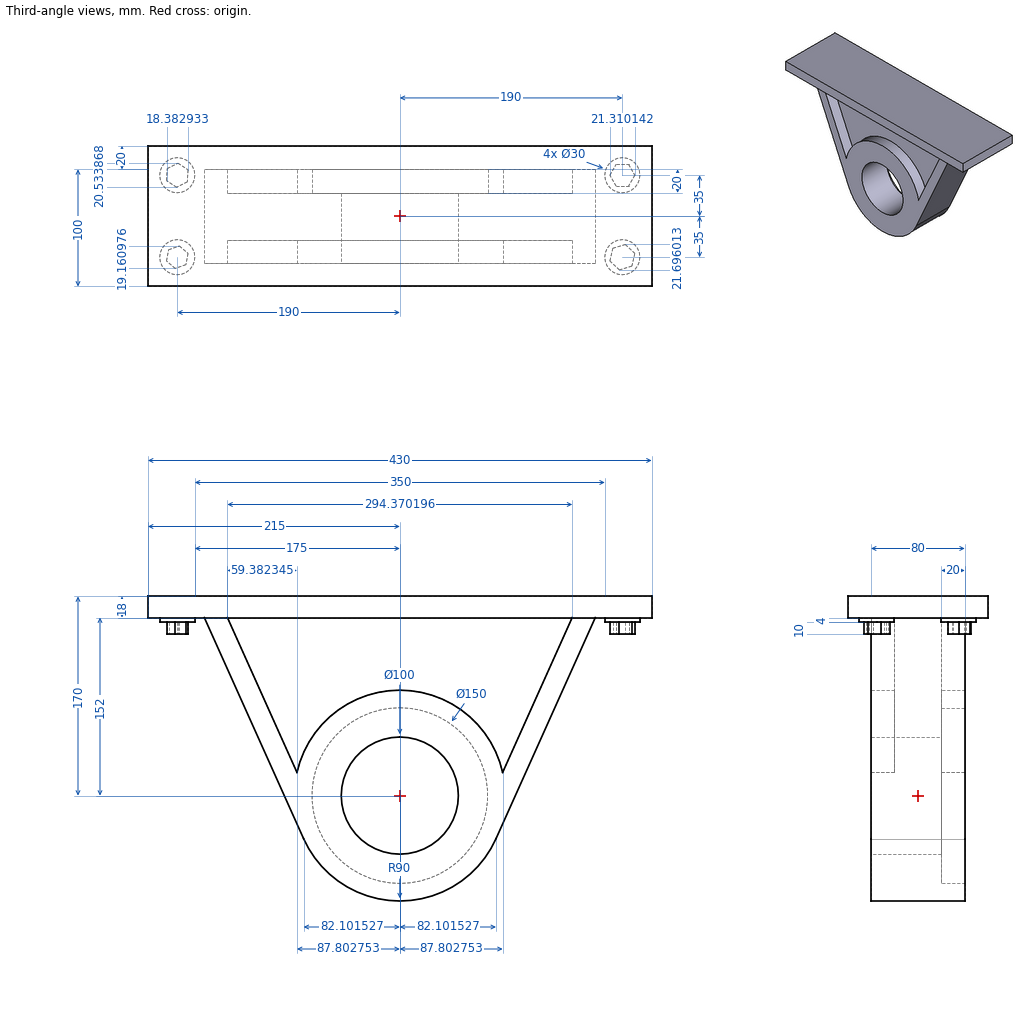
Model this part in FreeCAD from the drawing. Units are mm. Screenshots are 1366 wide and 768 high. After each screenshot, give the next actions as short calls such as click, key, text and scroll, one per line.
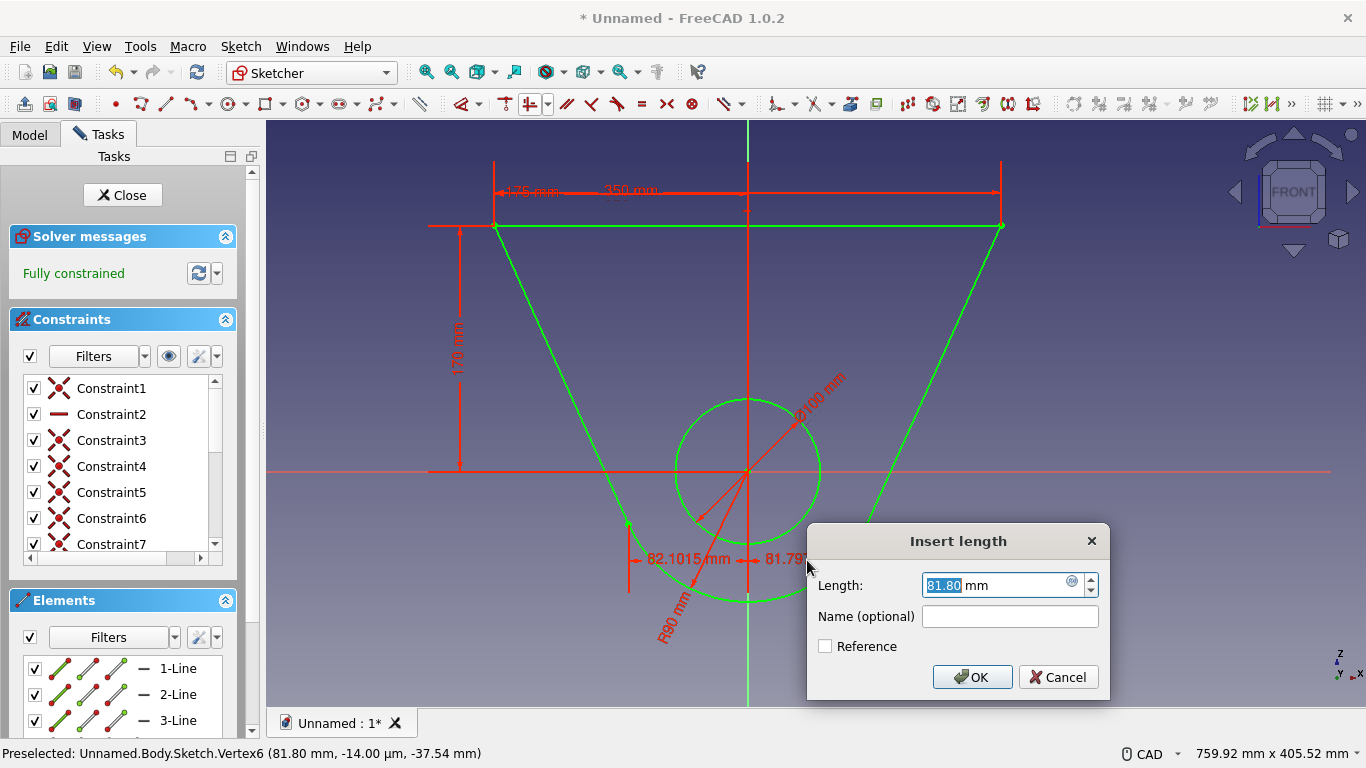
text(82.101527)
key(Return)
key(Escape)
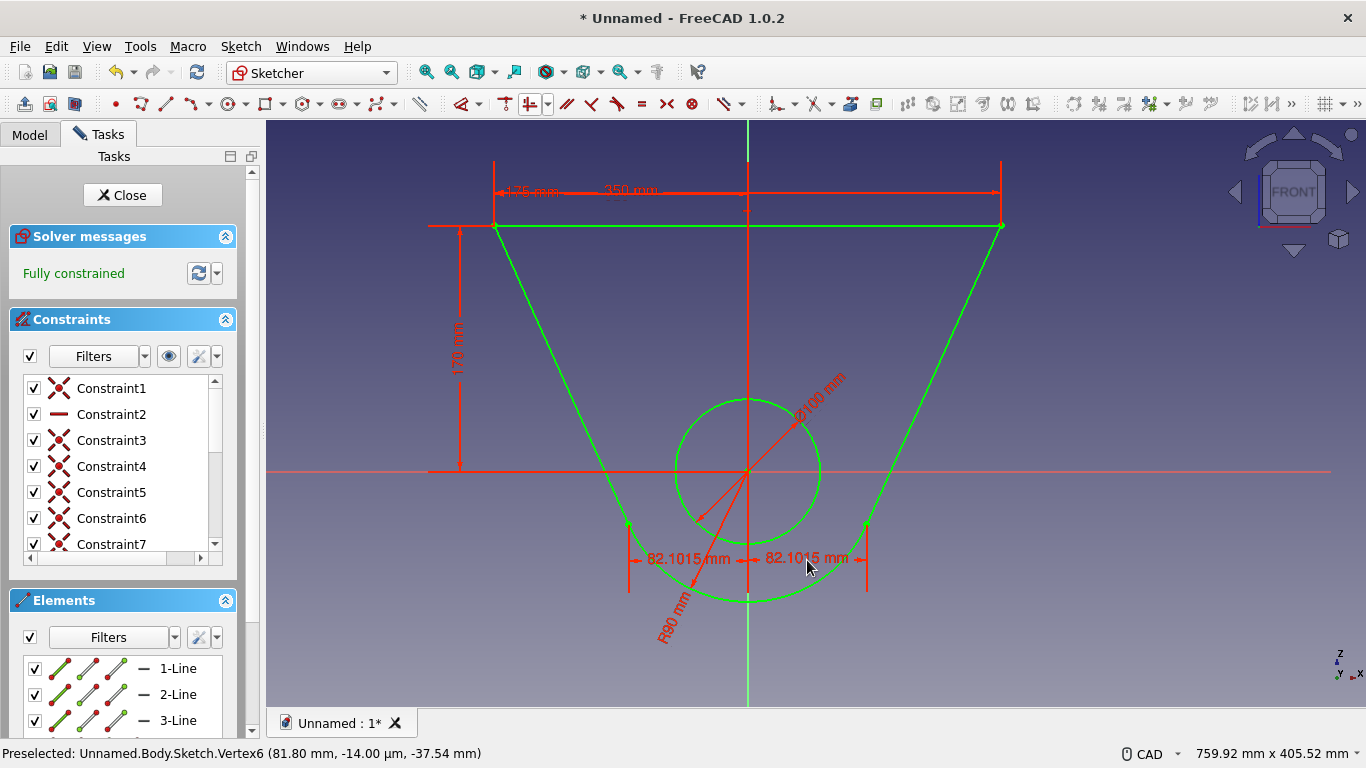
click(123, 195)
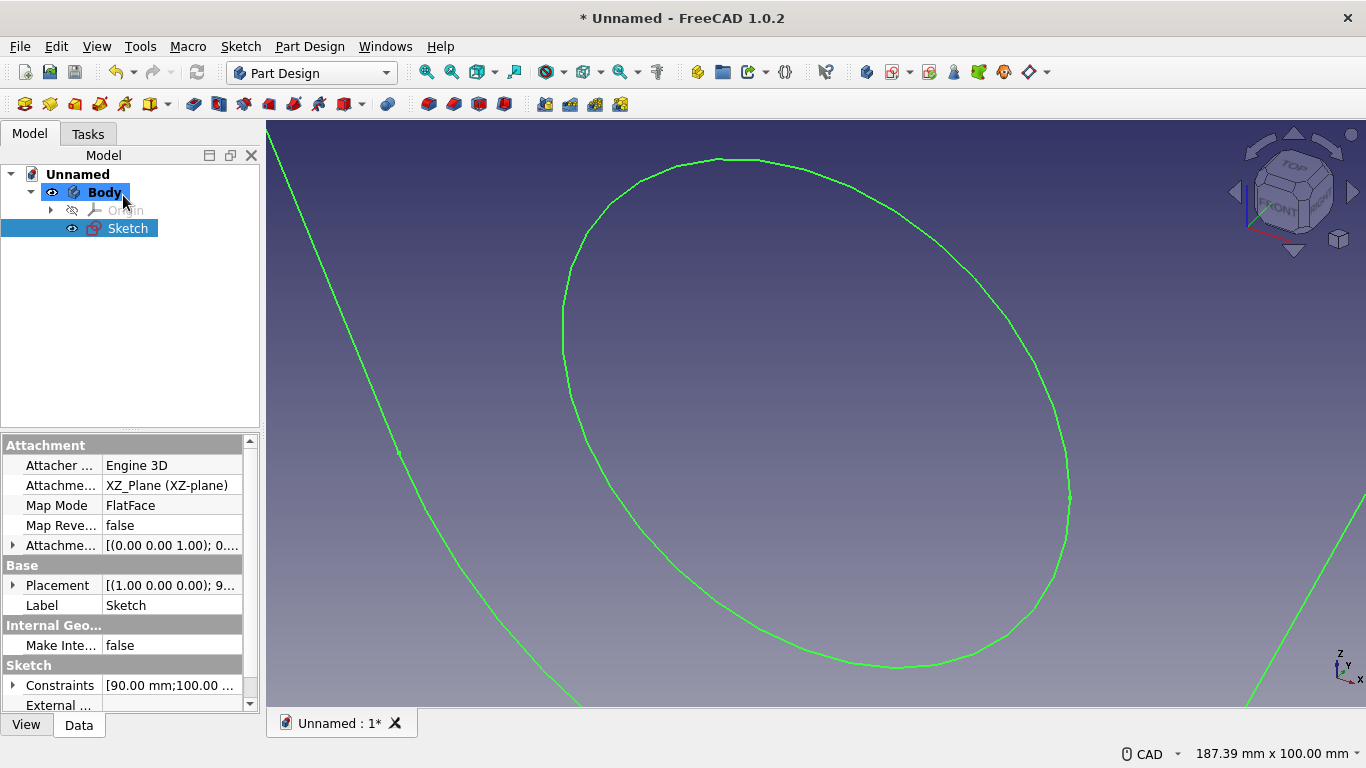
click(25, 104)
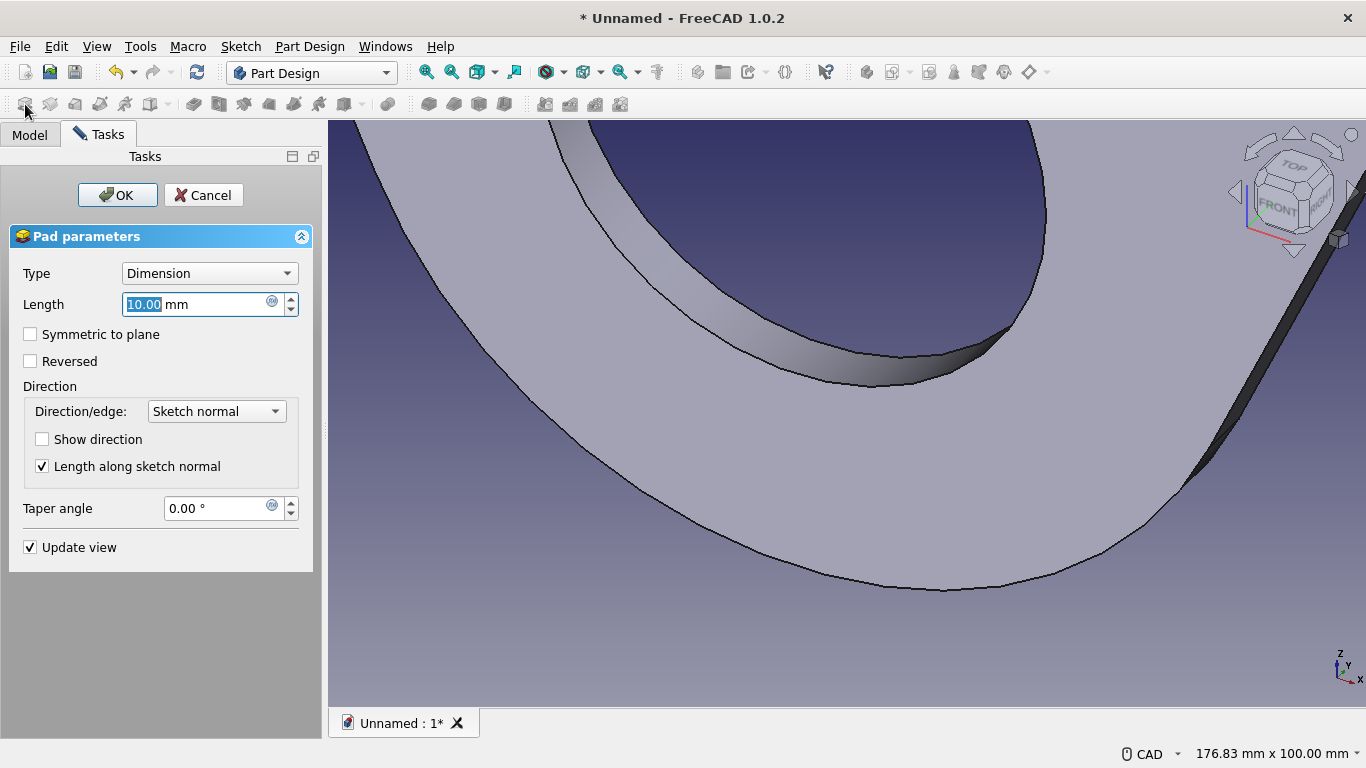
text(80)
key(Tab)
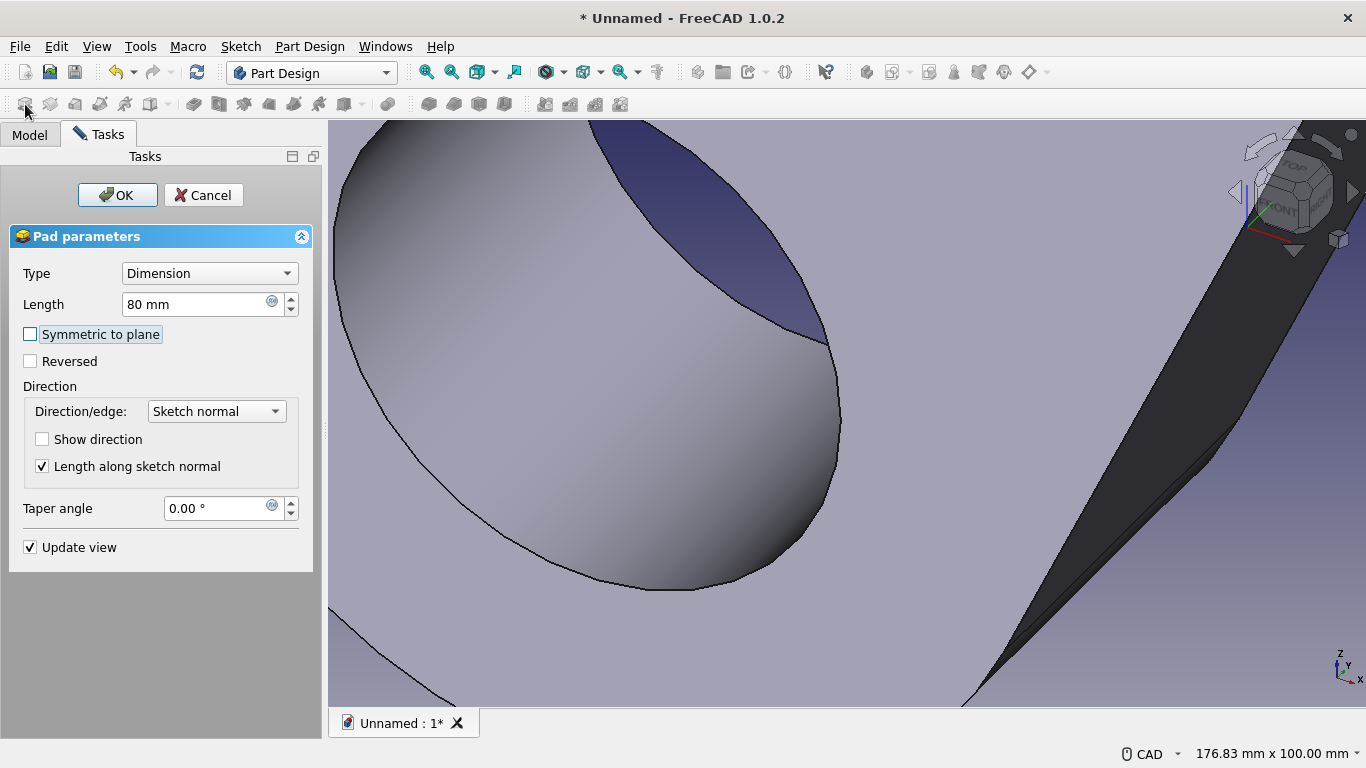
click(31, 334)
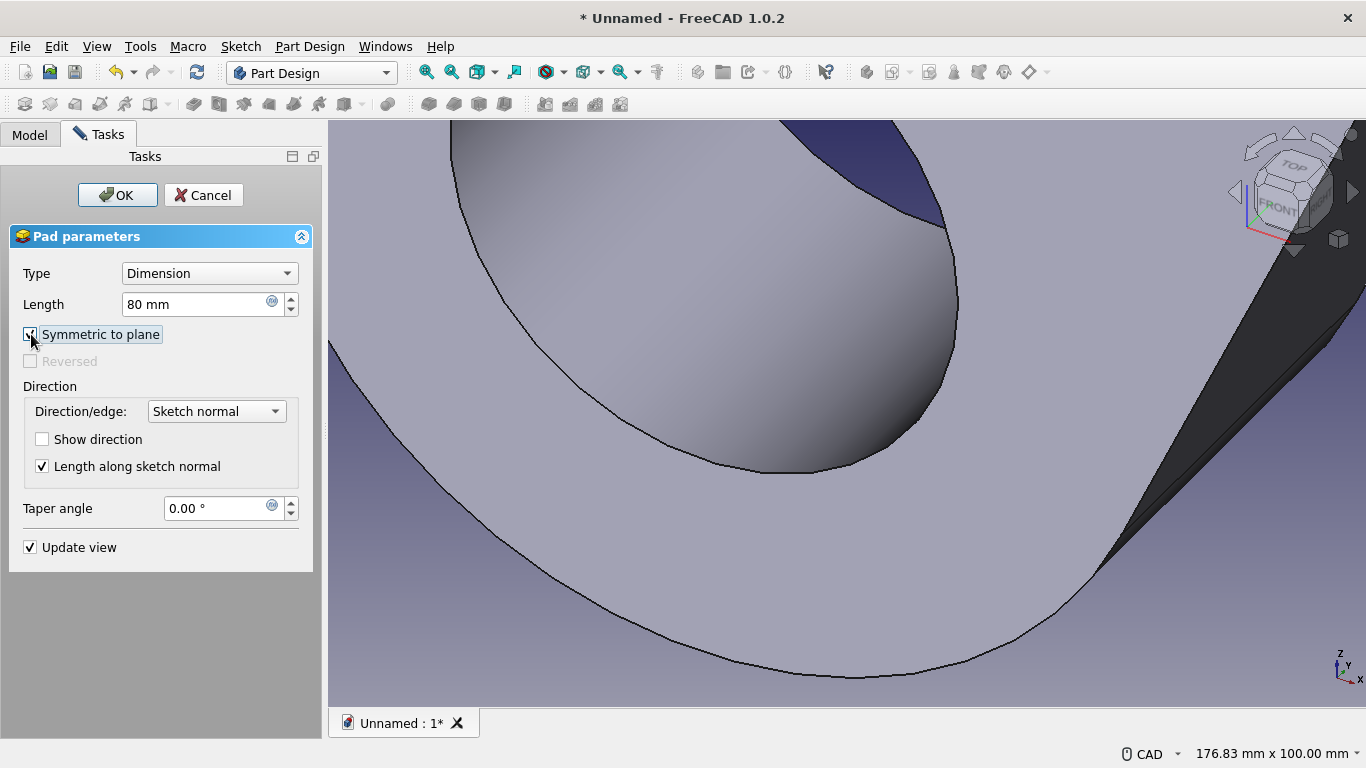
click(118, 195)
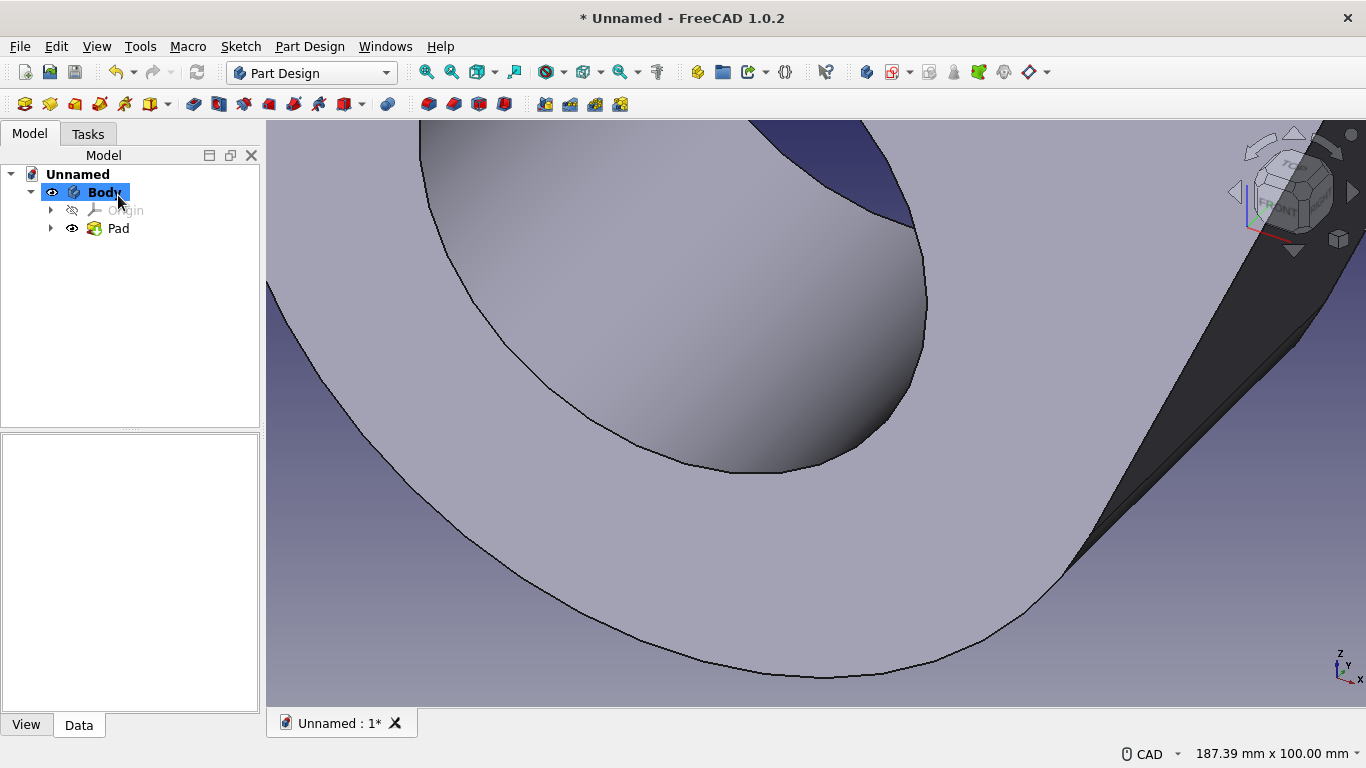
click(427, 72)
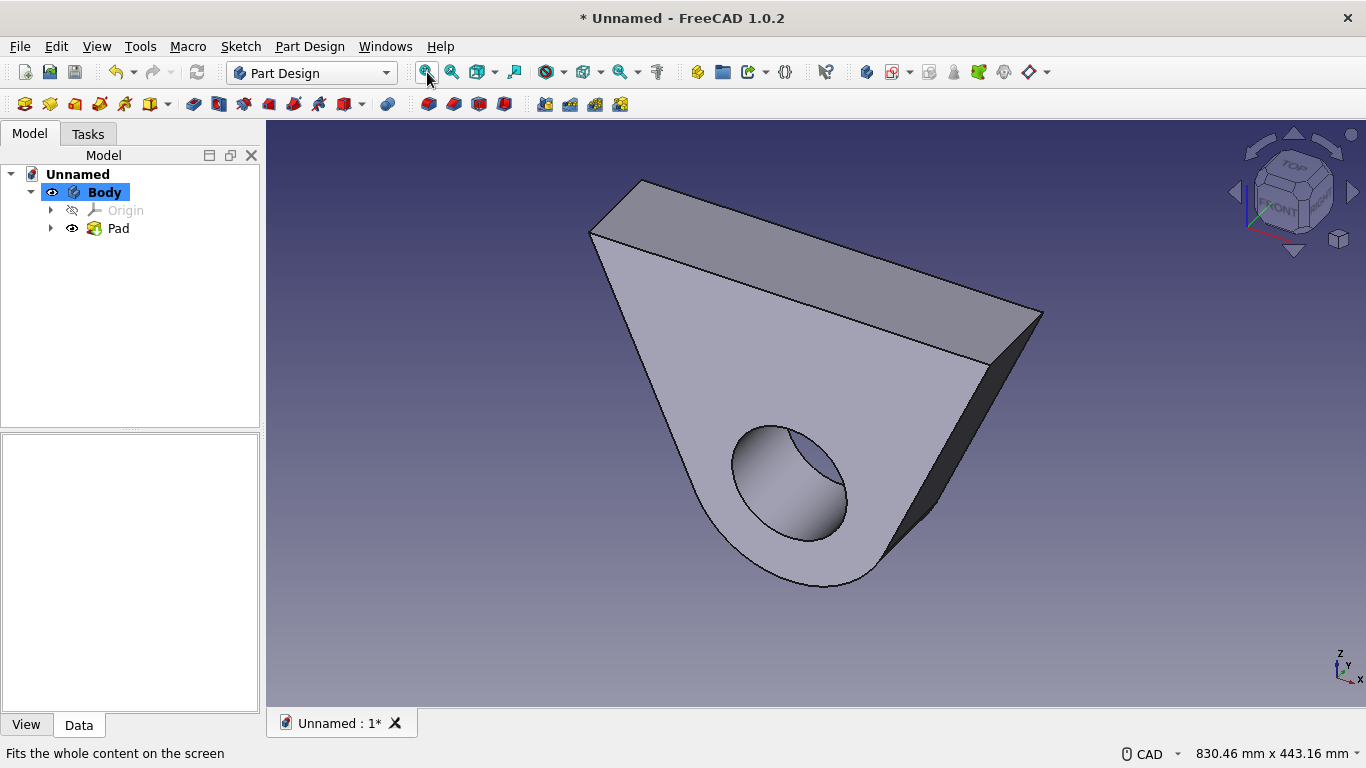
click(51, 210)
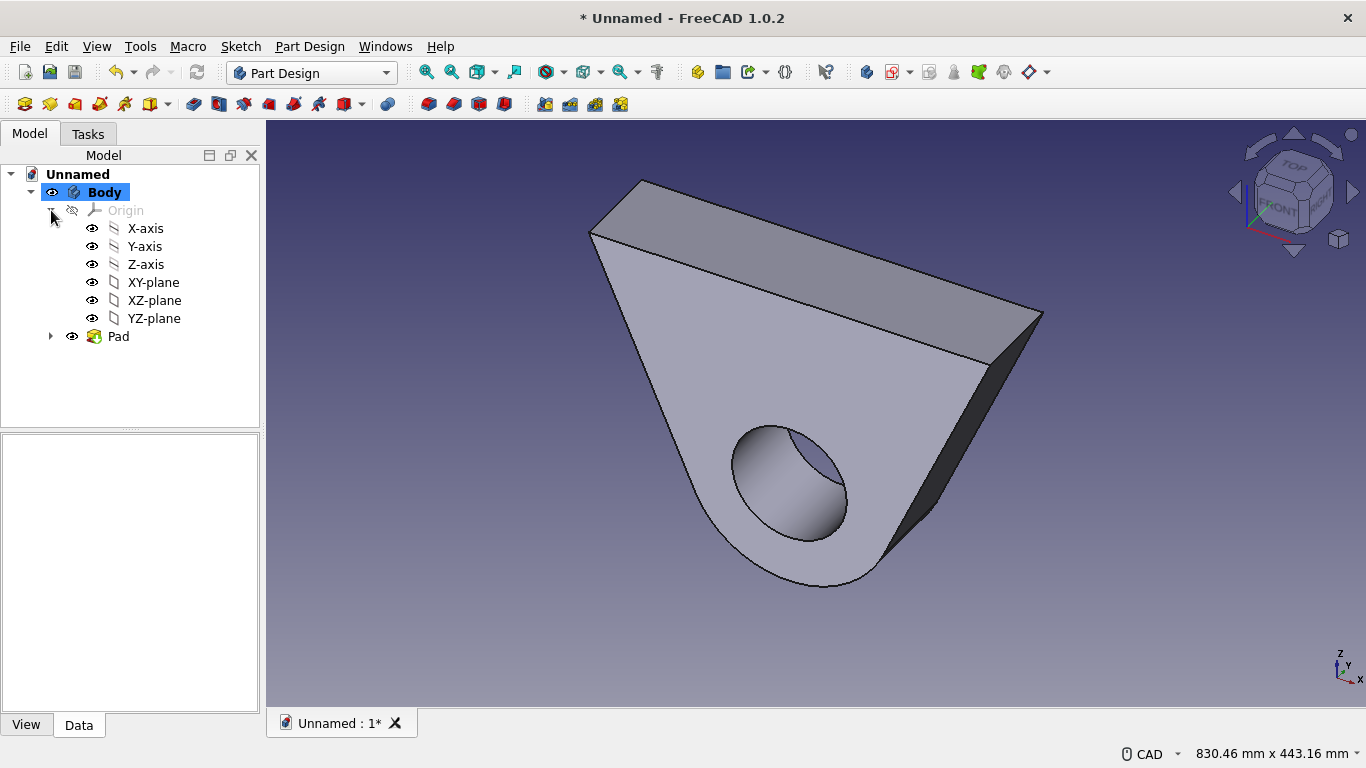
click(137, 300)